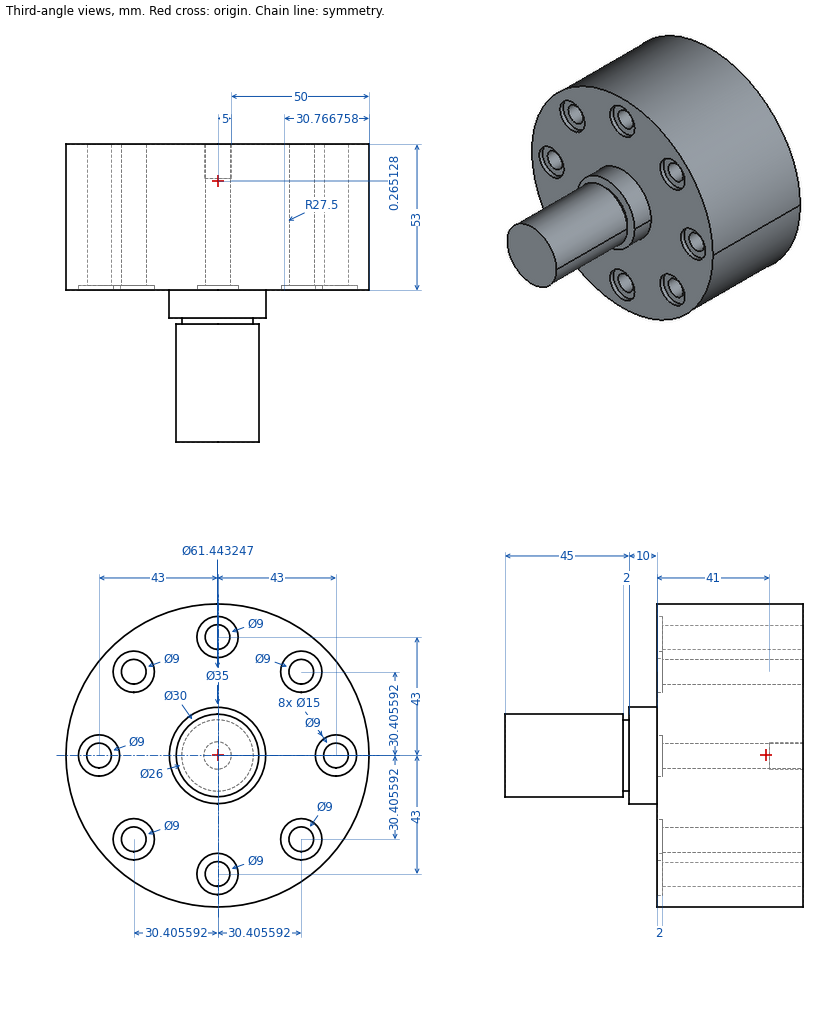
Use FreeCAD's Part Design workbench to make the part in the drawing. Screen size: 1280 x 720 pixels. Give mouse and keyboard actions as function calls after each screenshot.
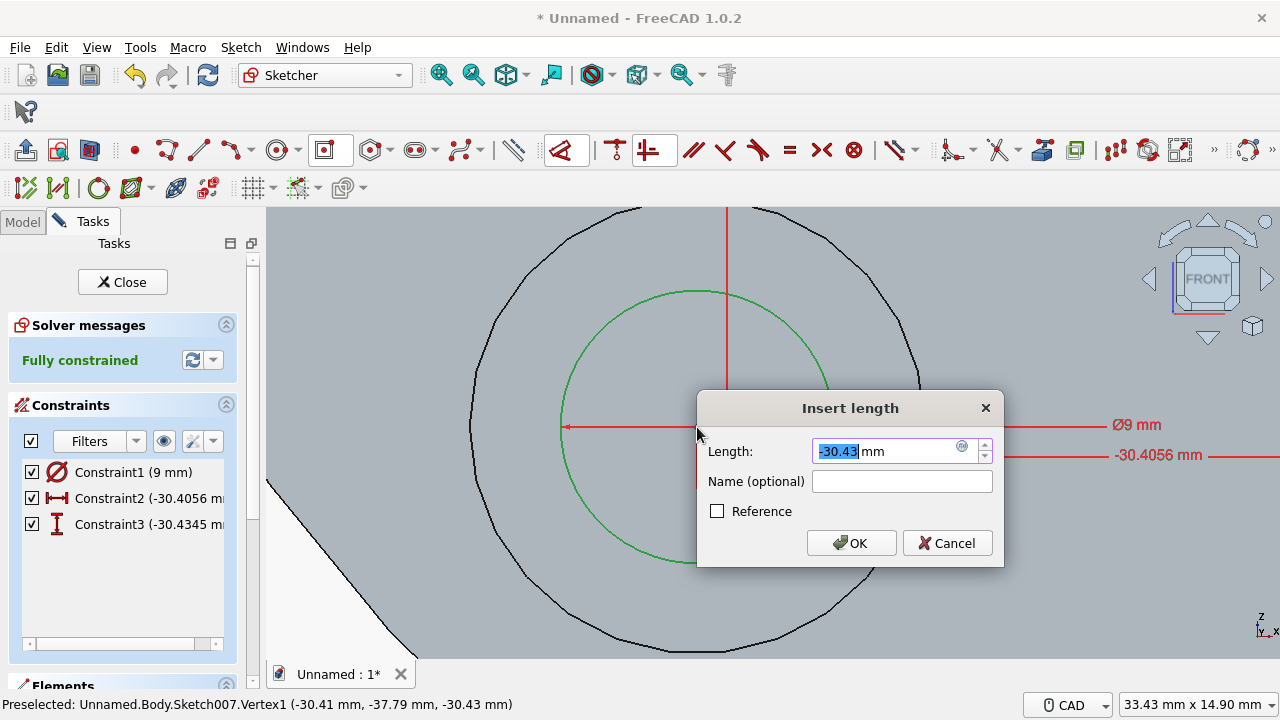
text(-30.405592)
key(Return)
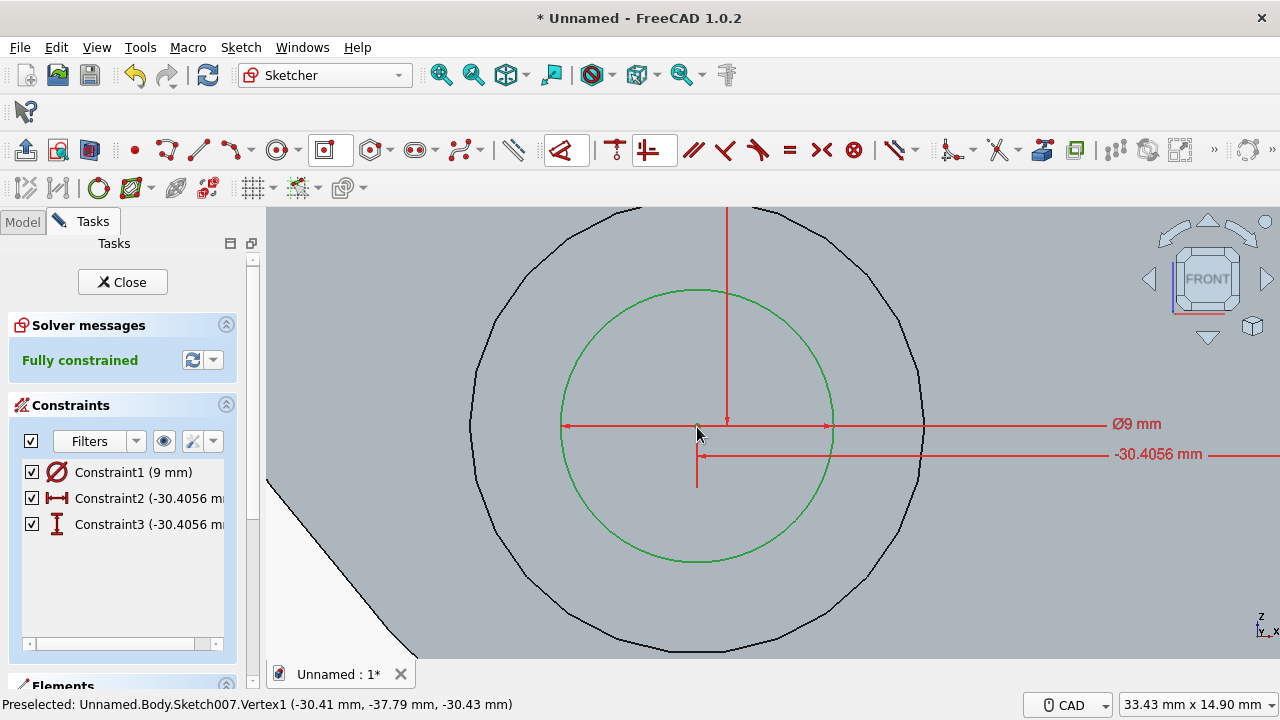
click(123, 282)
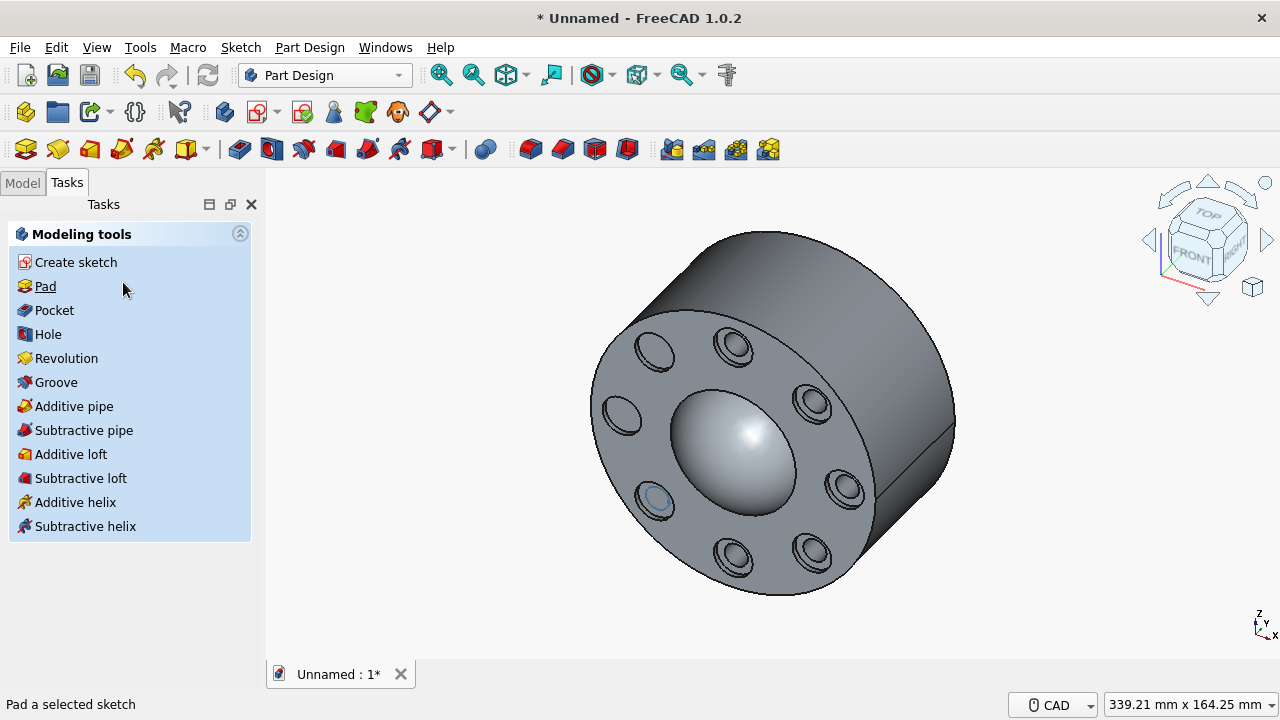
click(240, 150)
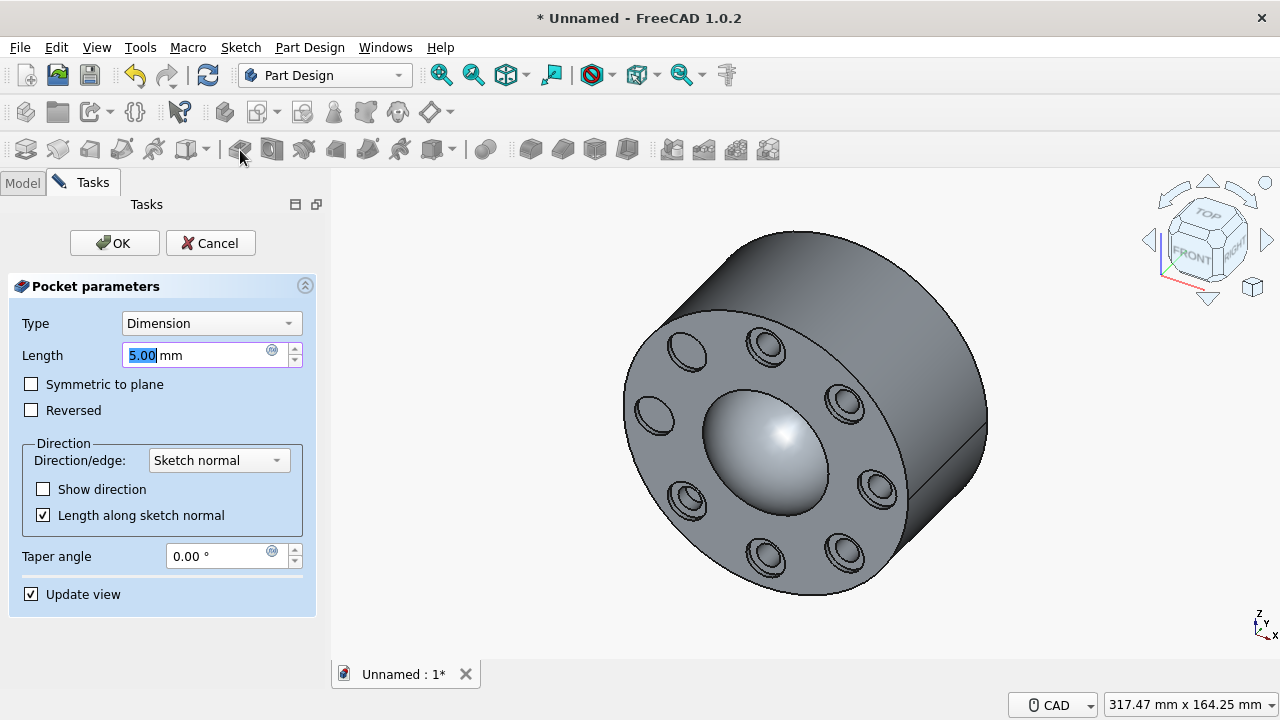
click(212, 324)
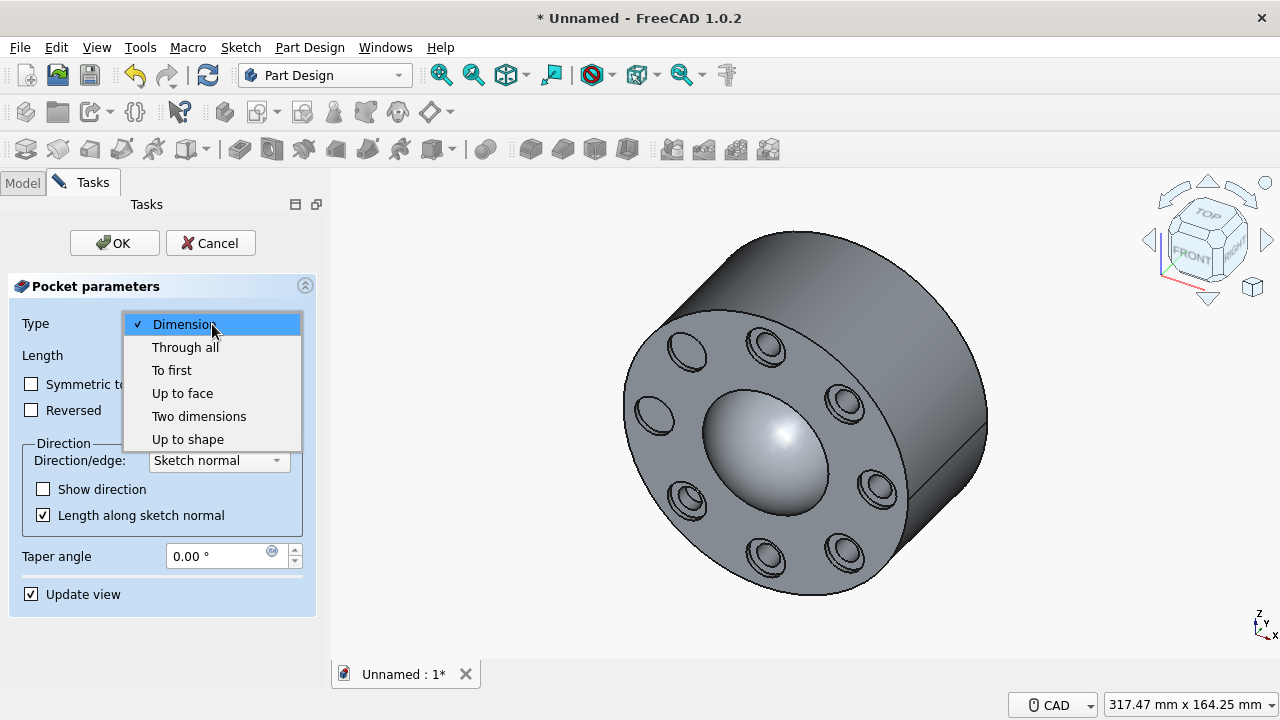
click(212, 370)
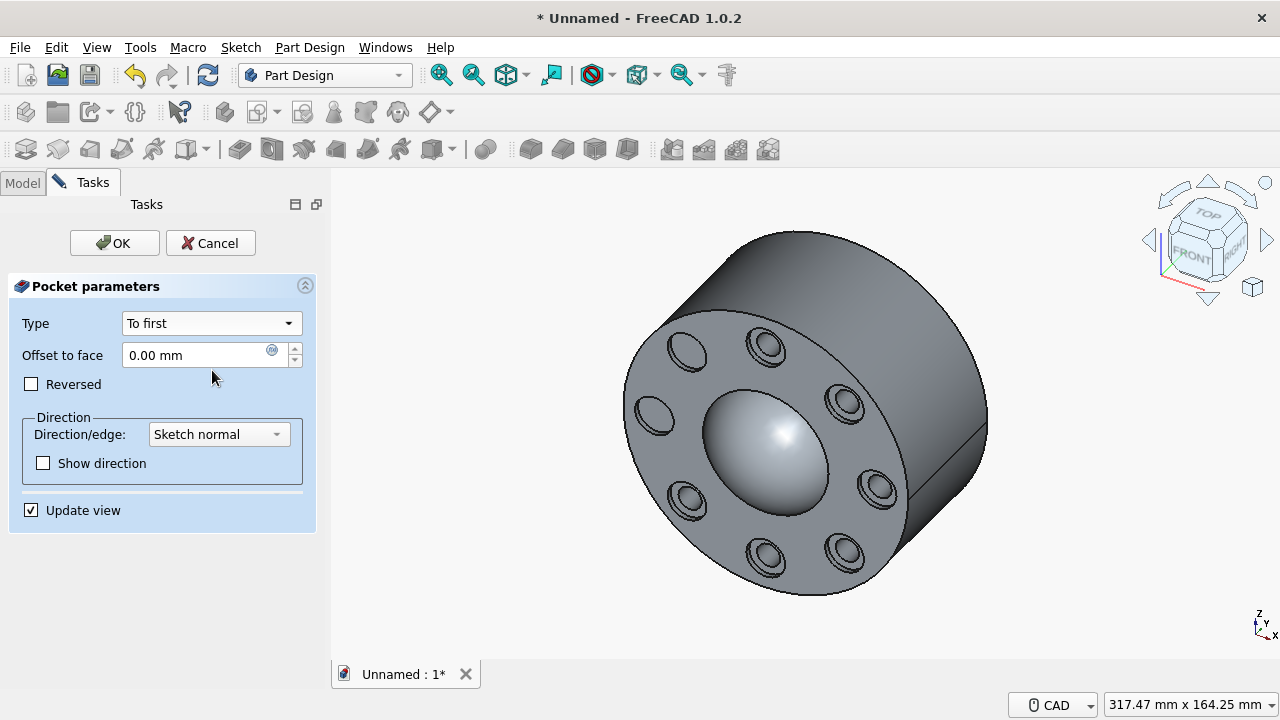
click(115, 243)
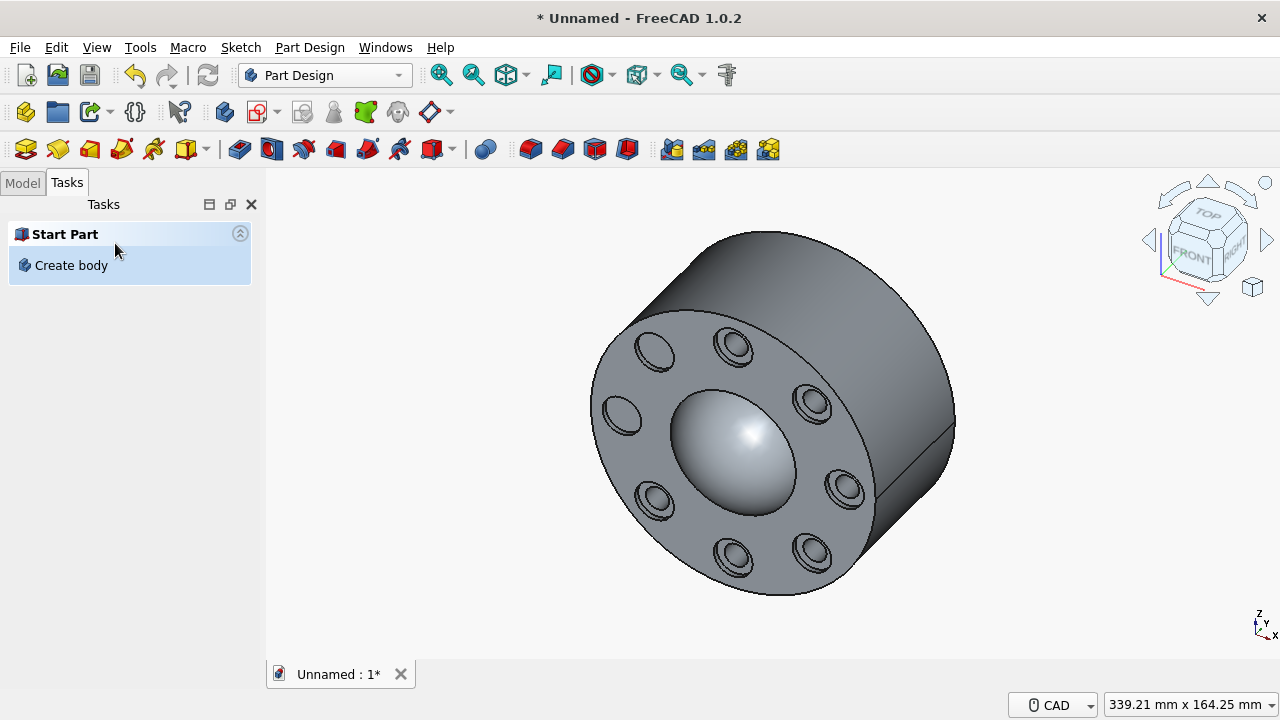
click(658, 348)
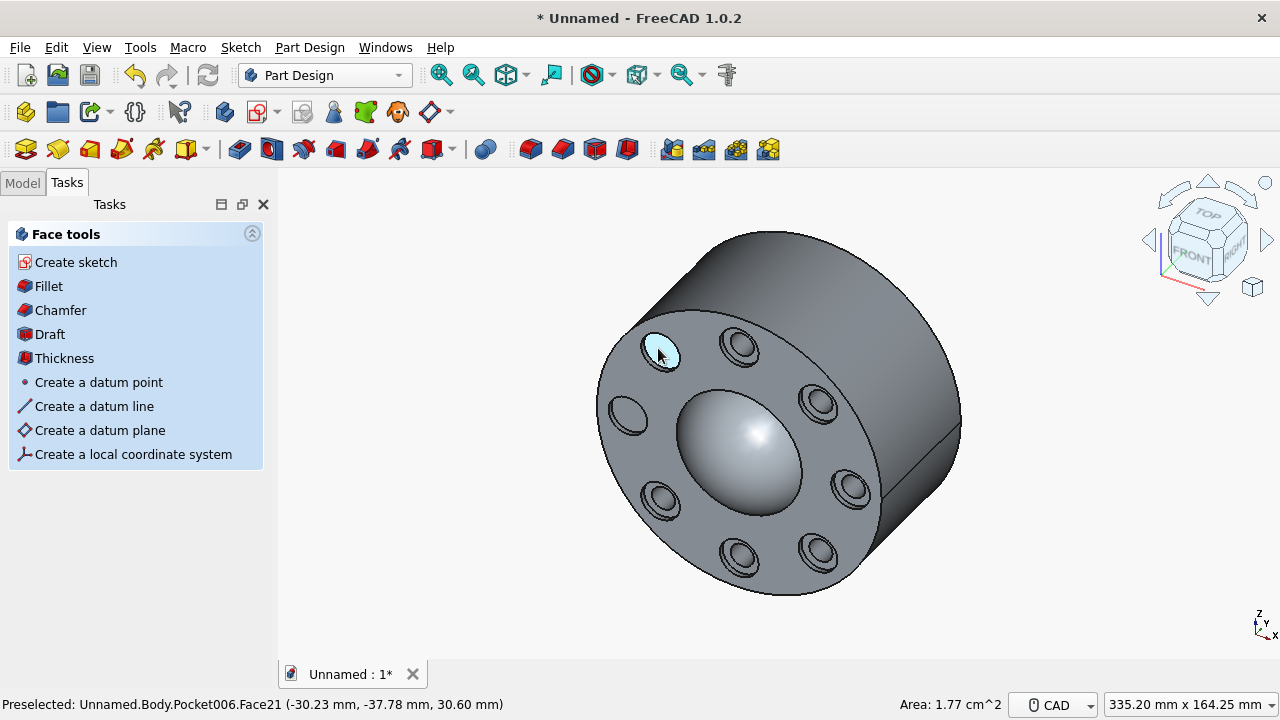
click(258, 112)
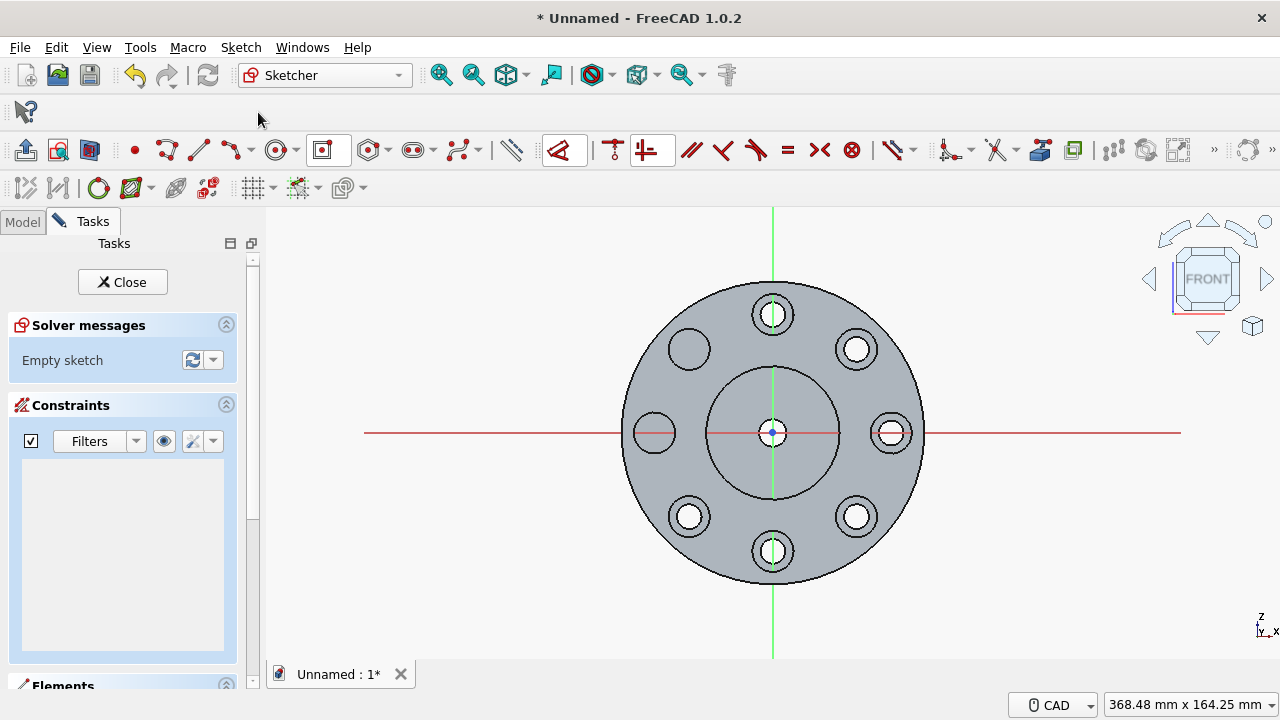
click(90, 150)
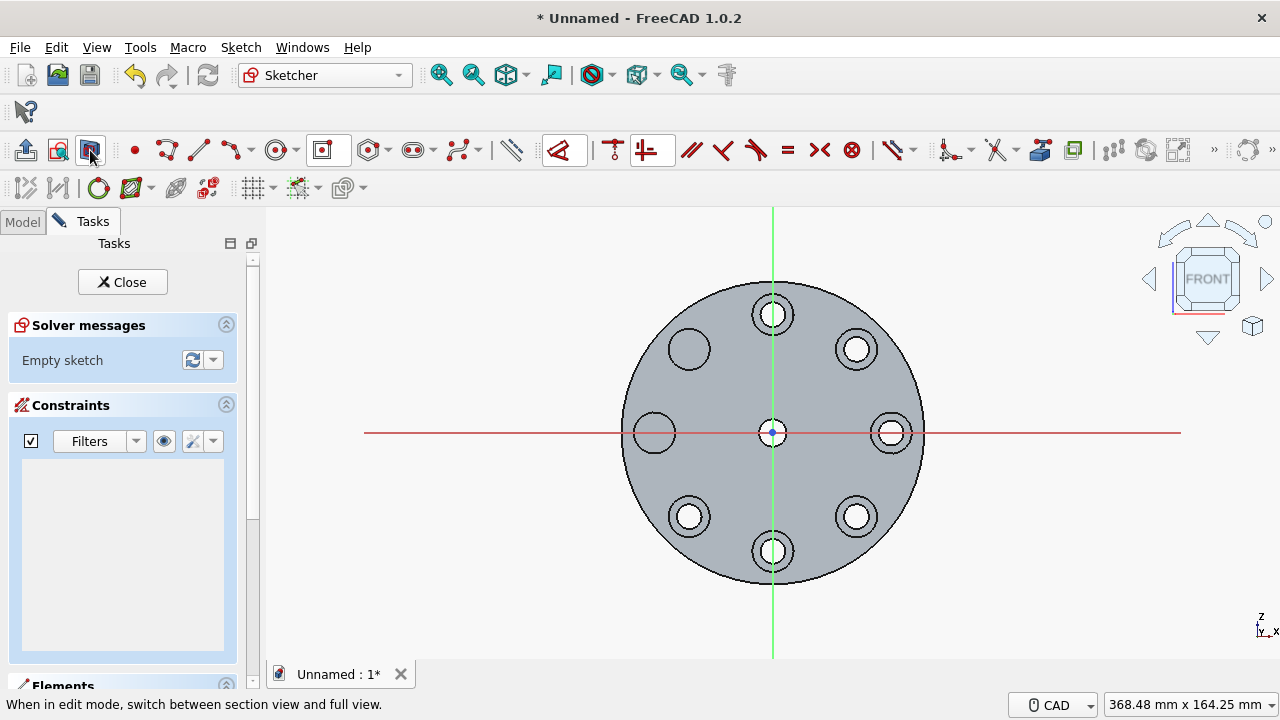
scroll(650, 433, up, 12)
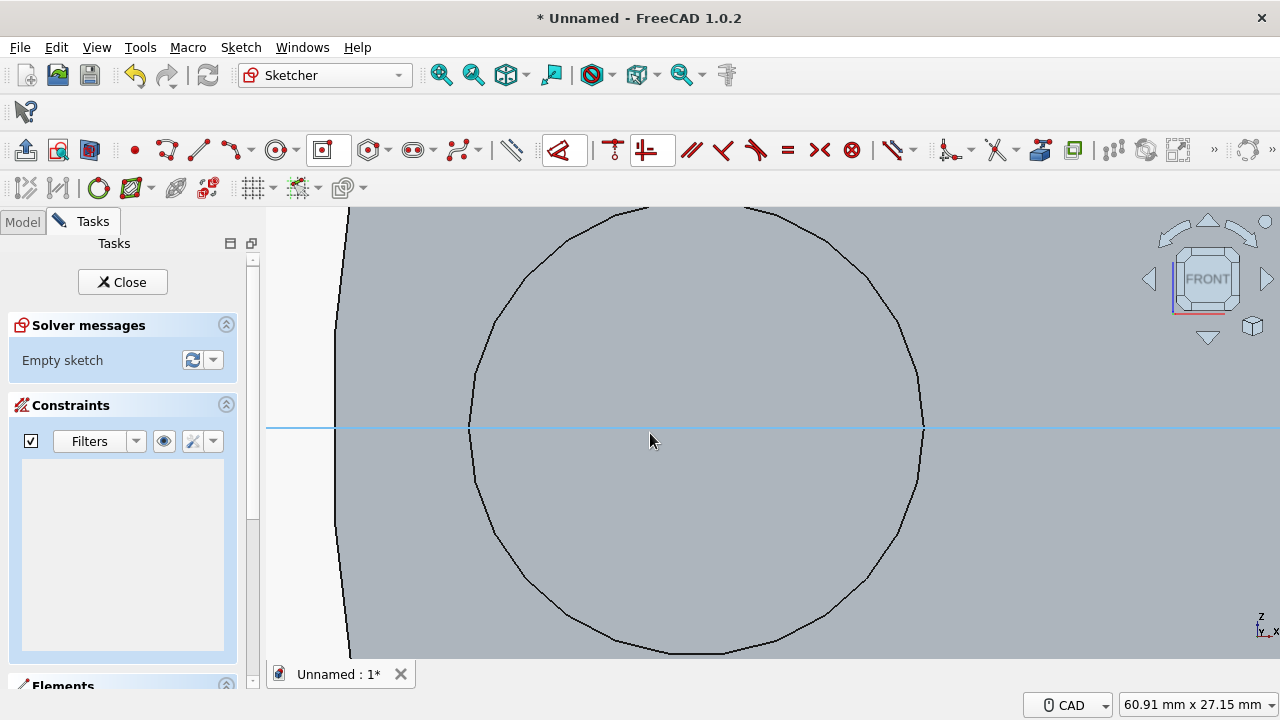
click(276, 150)